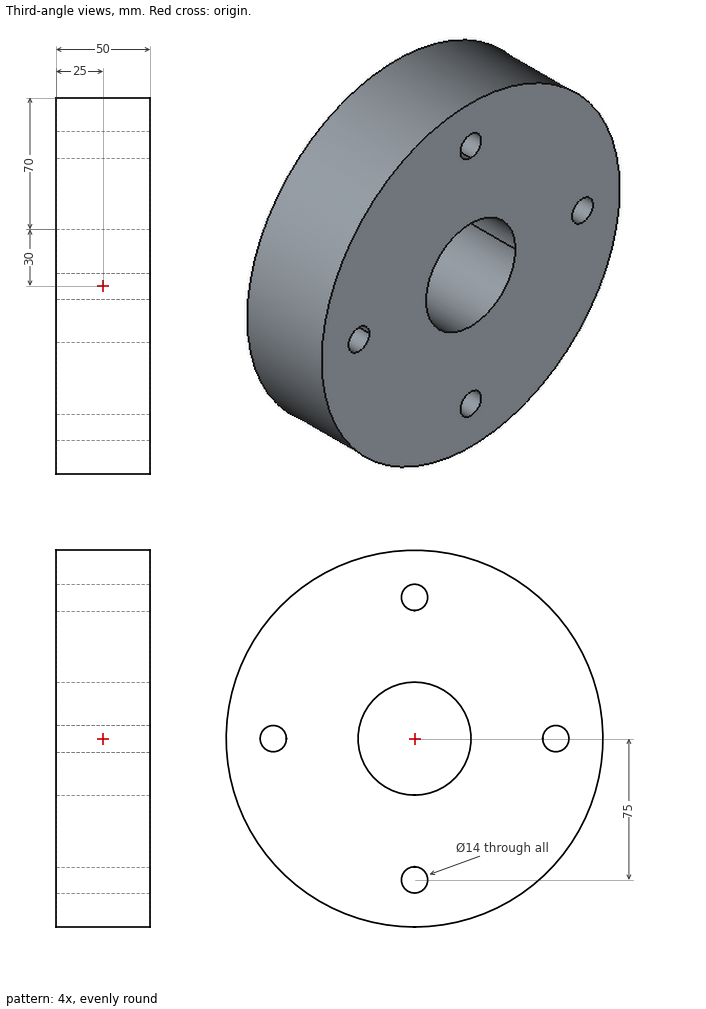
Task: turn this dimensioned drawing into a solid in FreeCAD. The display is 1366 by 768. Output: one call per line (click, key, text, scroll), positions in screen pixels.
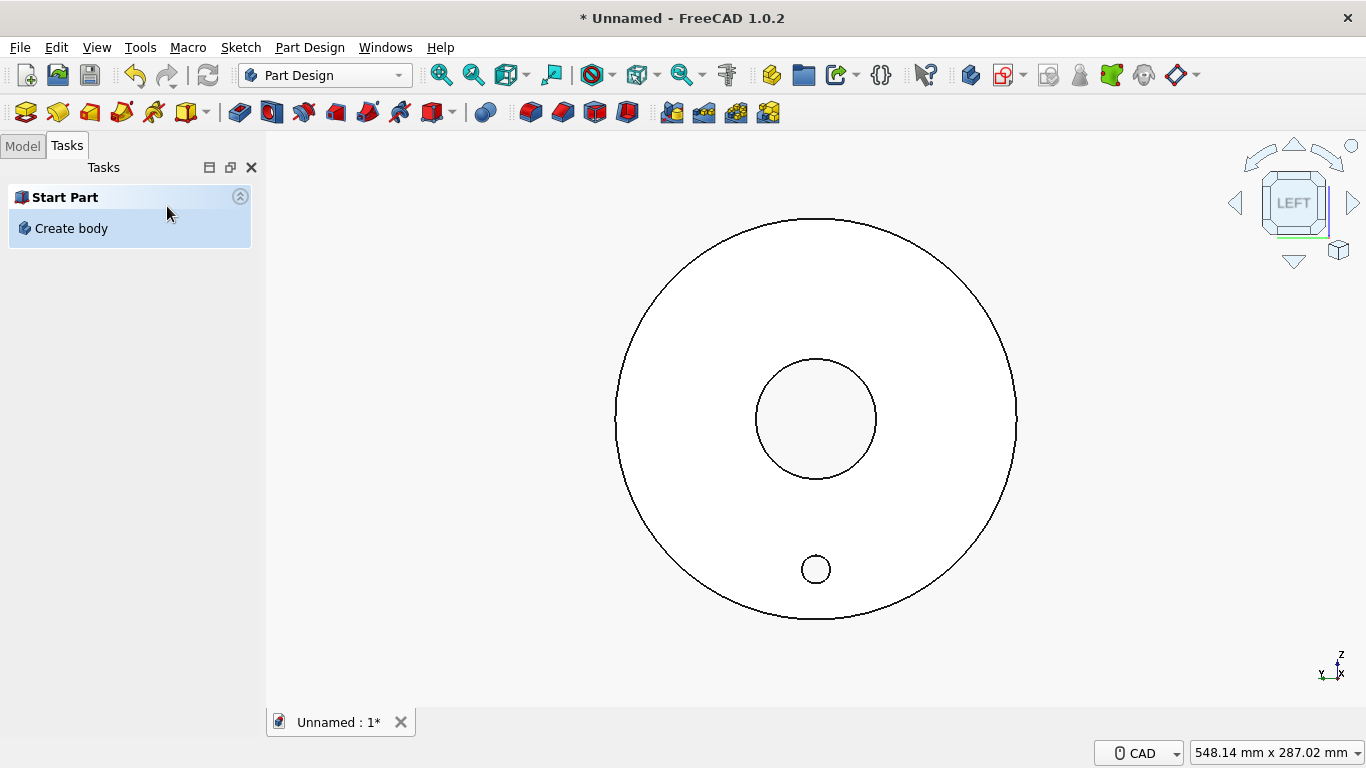
click(23, 145)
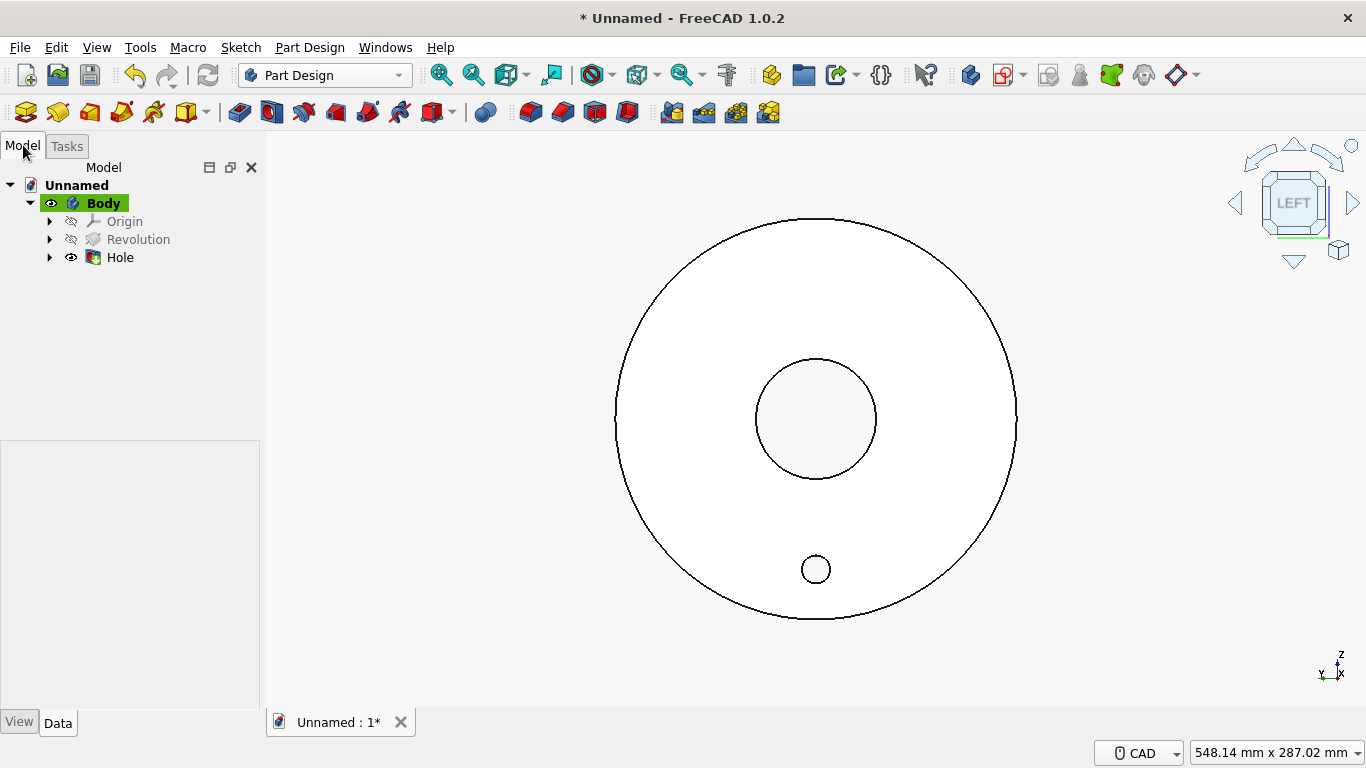
click(116, 257)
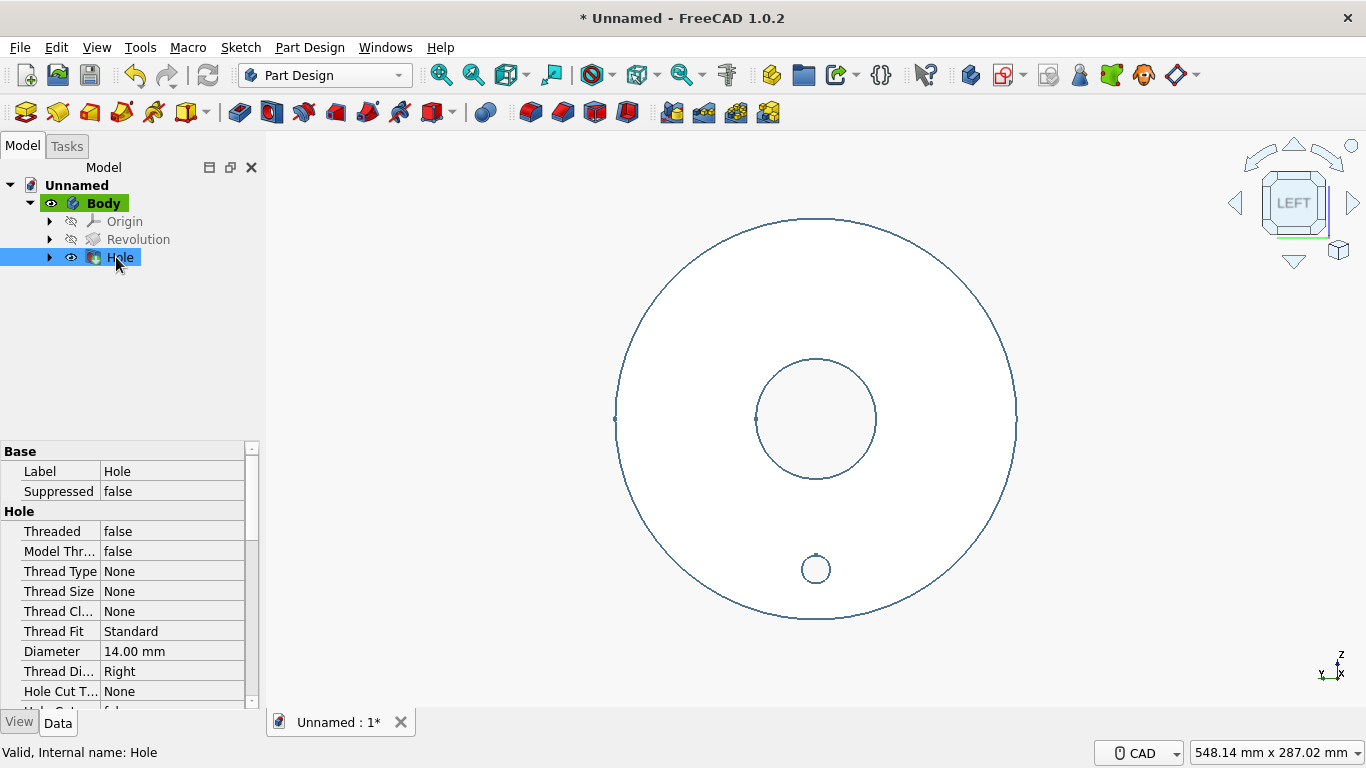
click(736, 112)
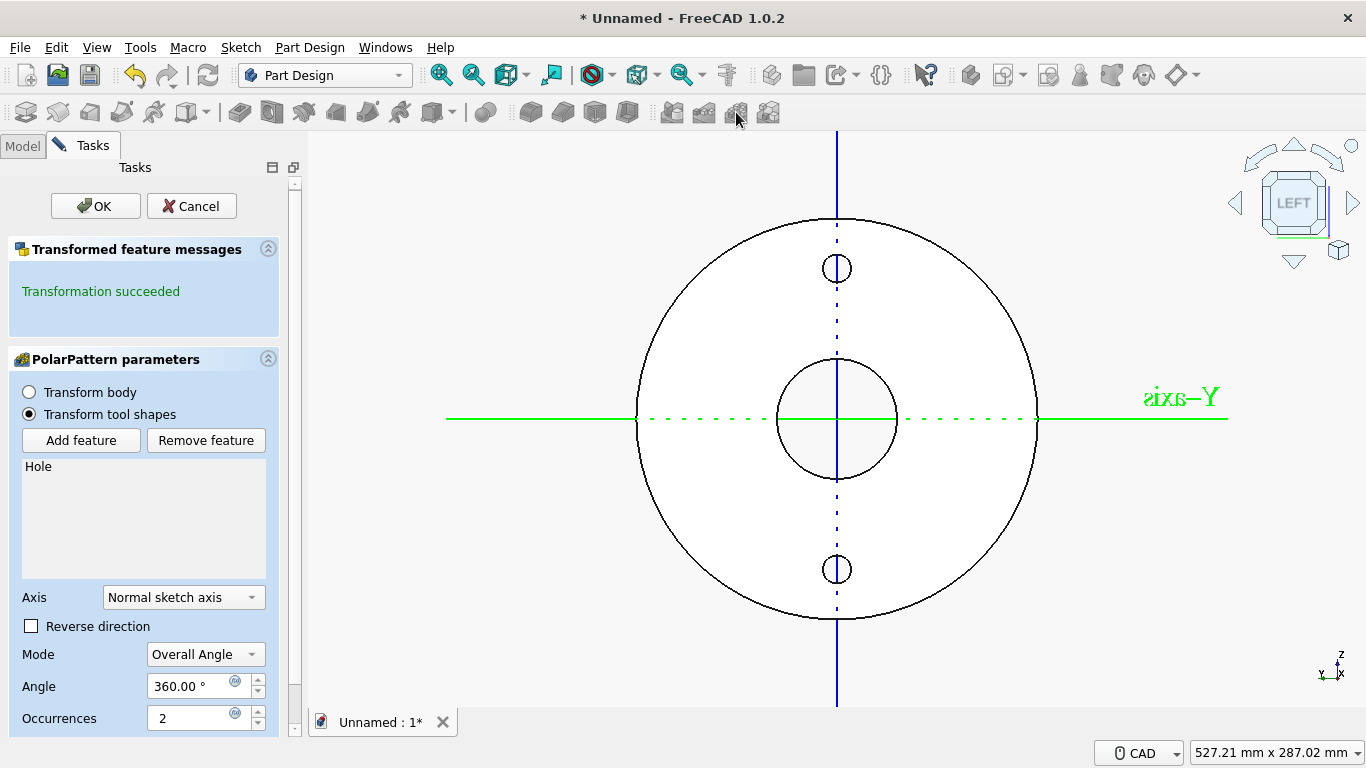
click(184, 598)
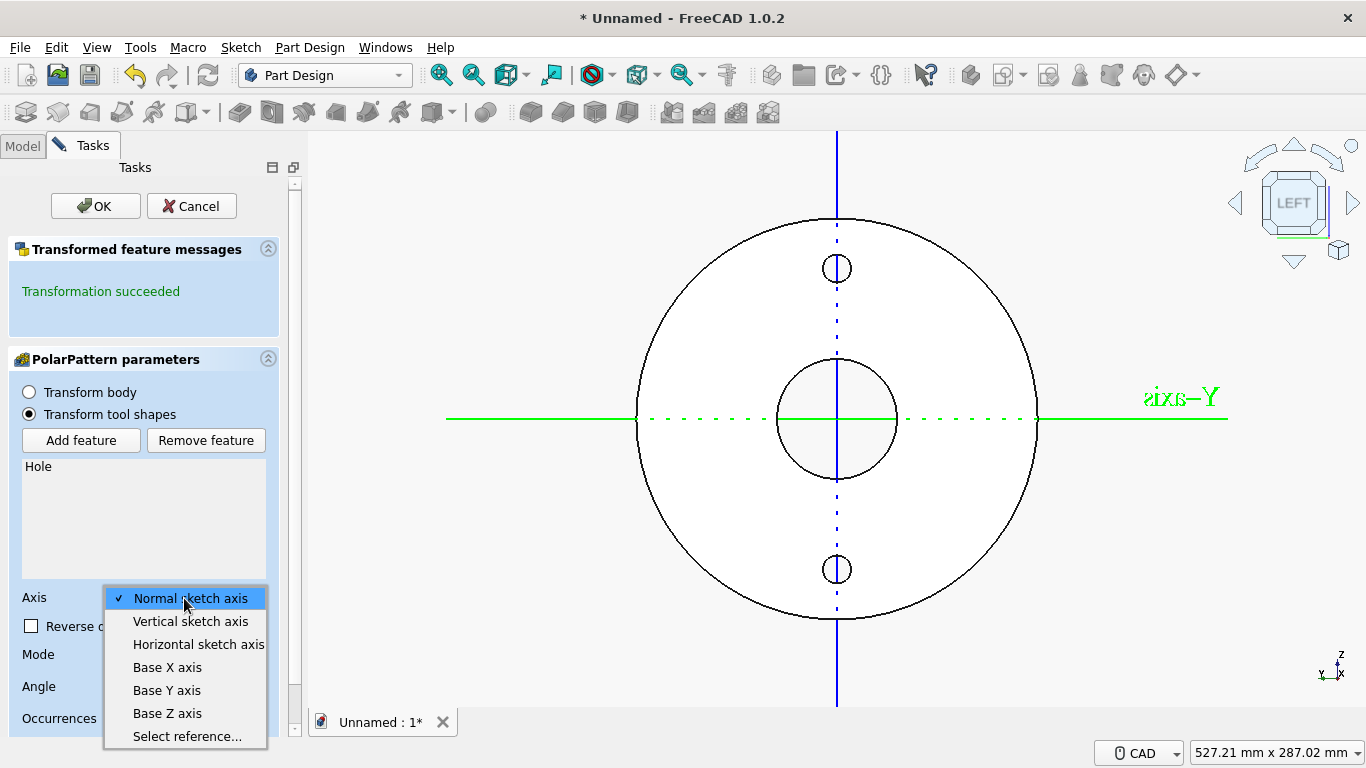
click(184, 668)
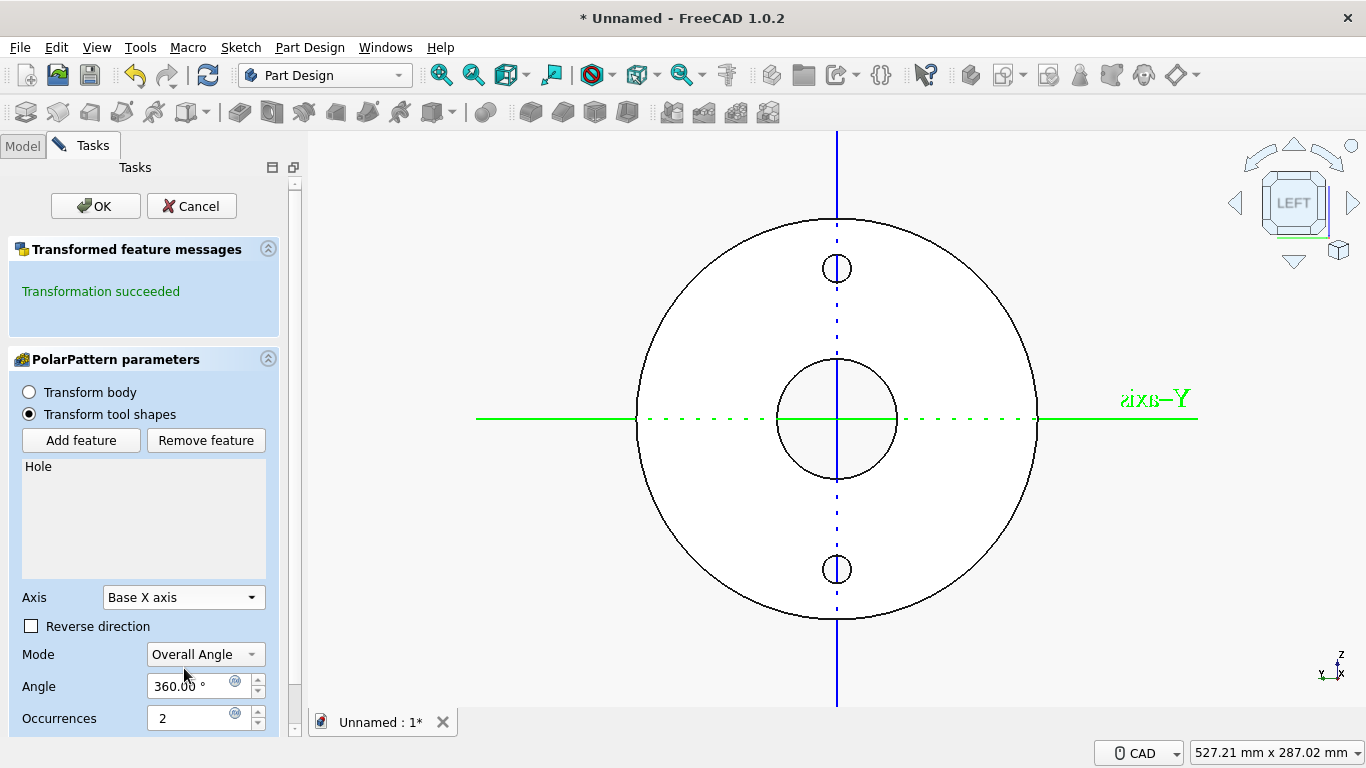
triple_click(198, 718)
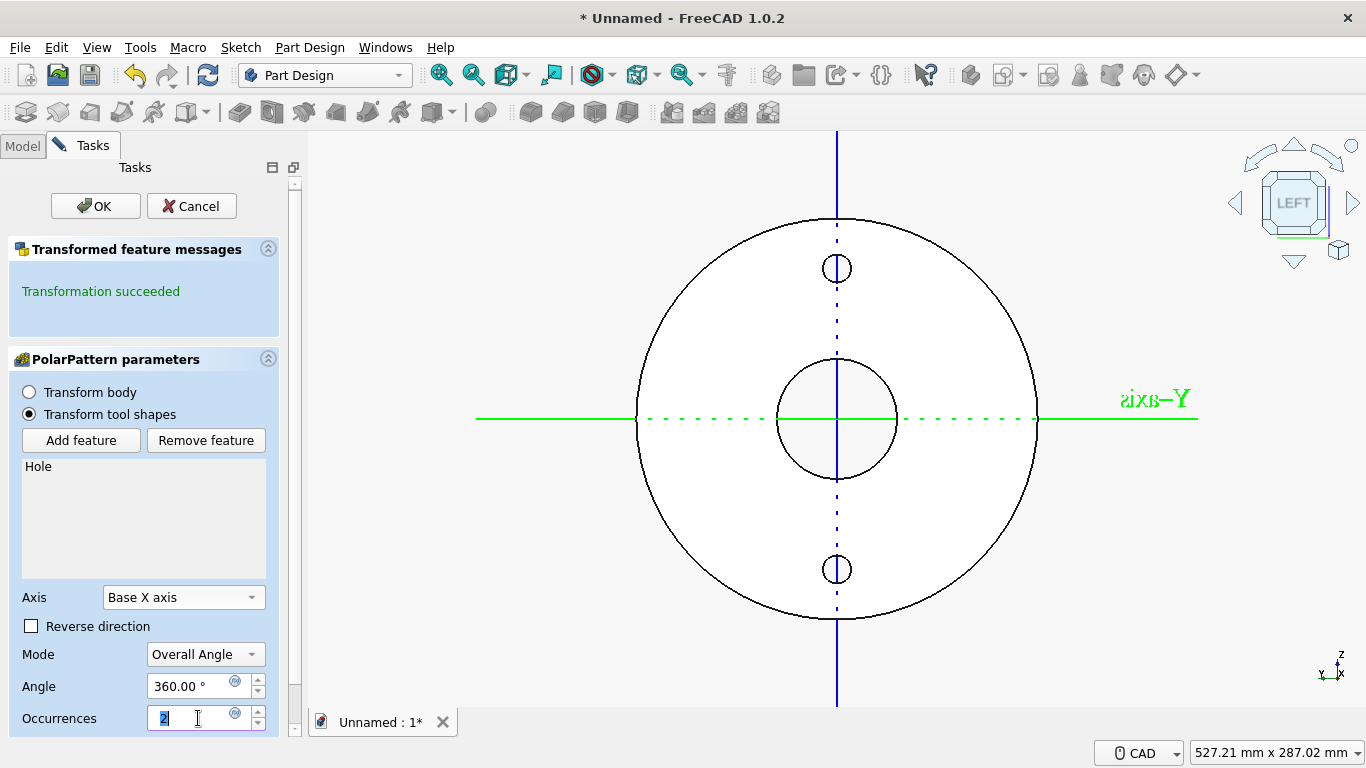
text(4)
key(Tab)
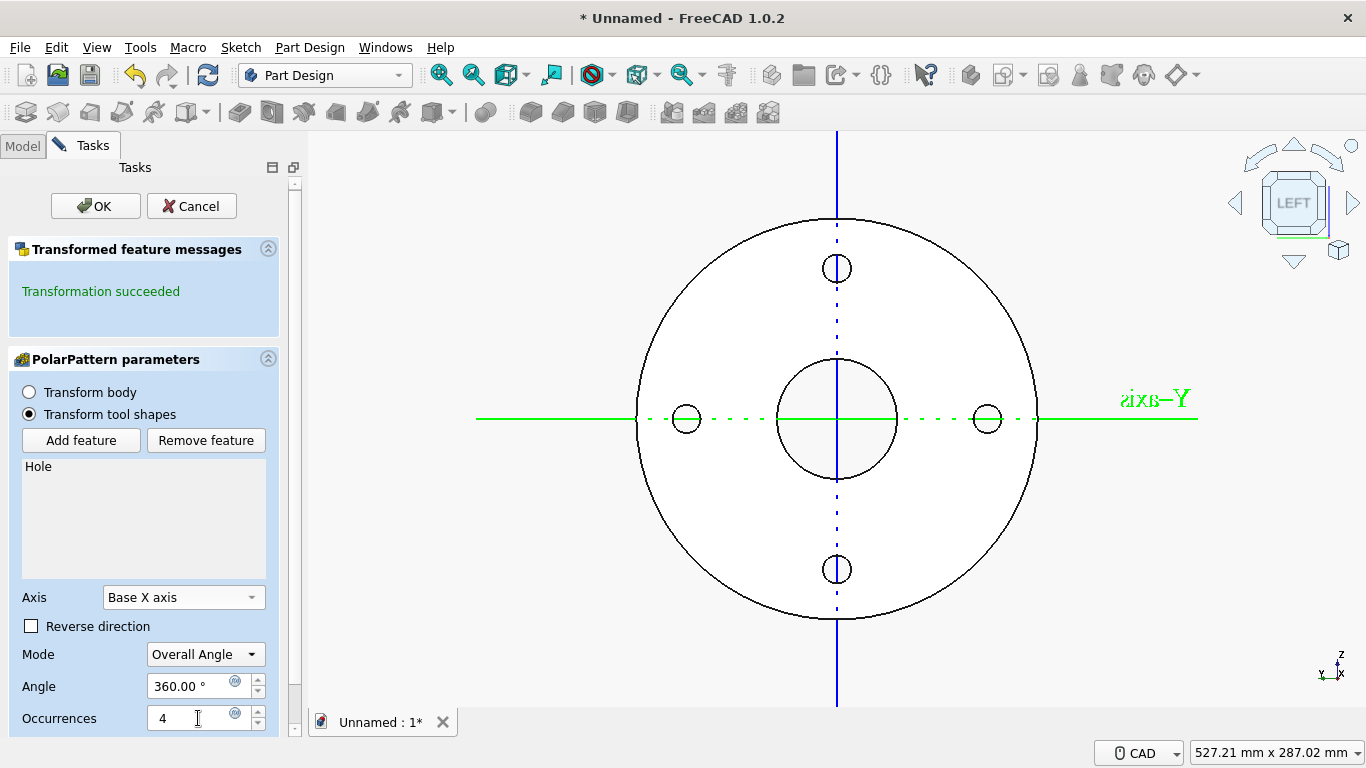
click(96, 206)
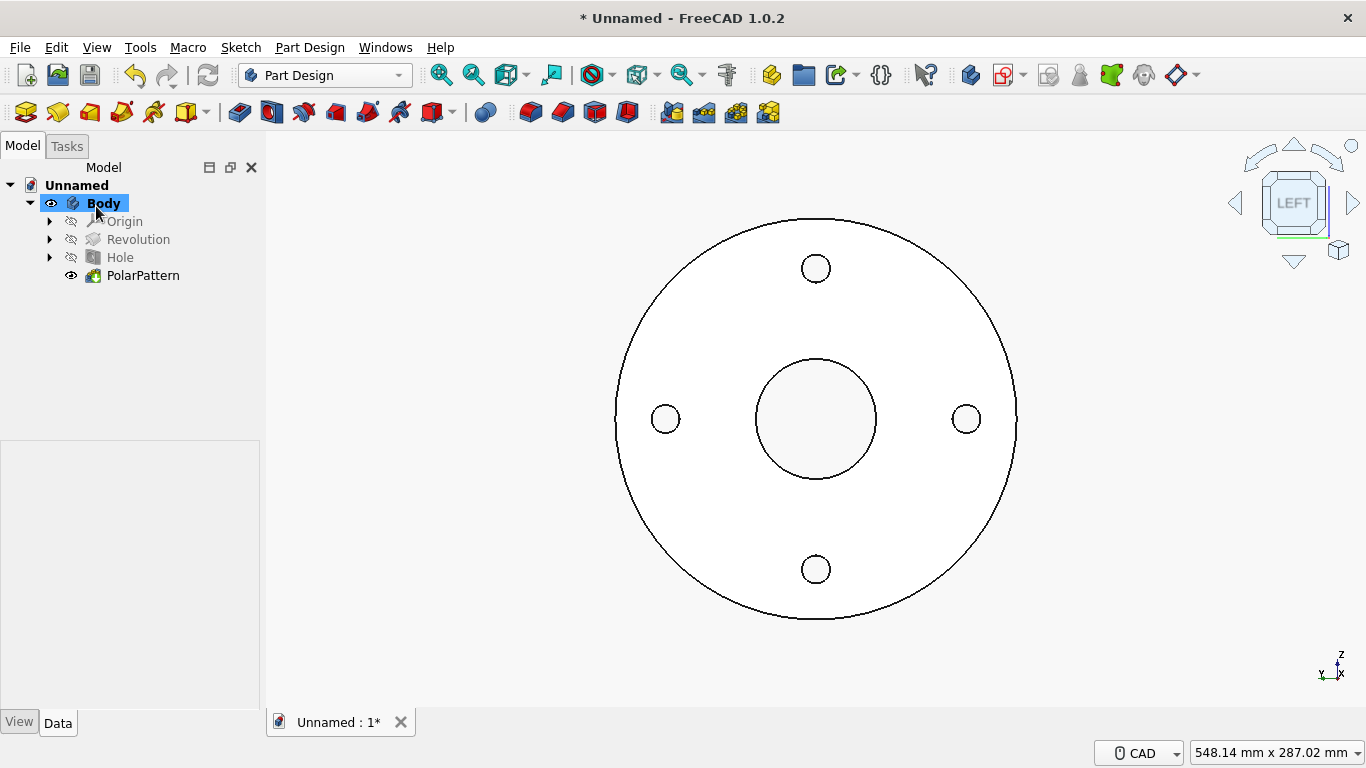
key(0)